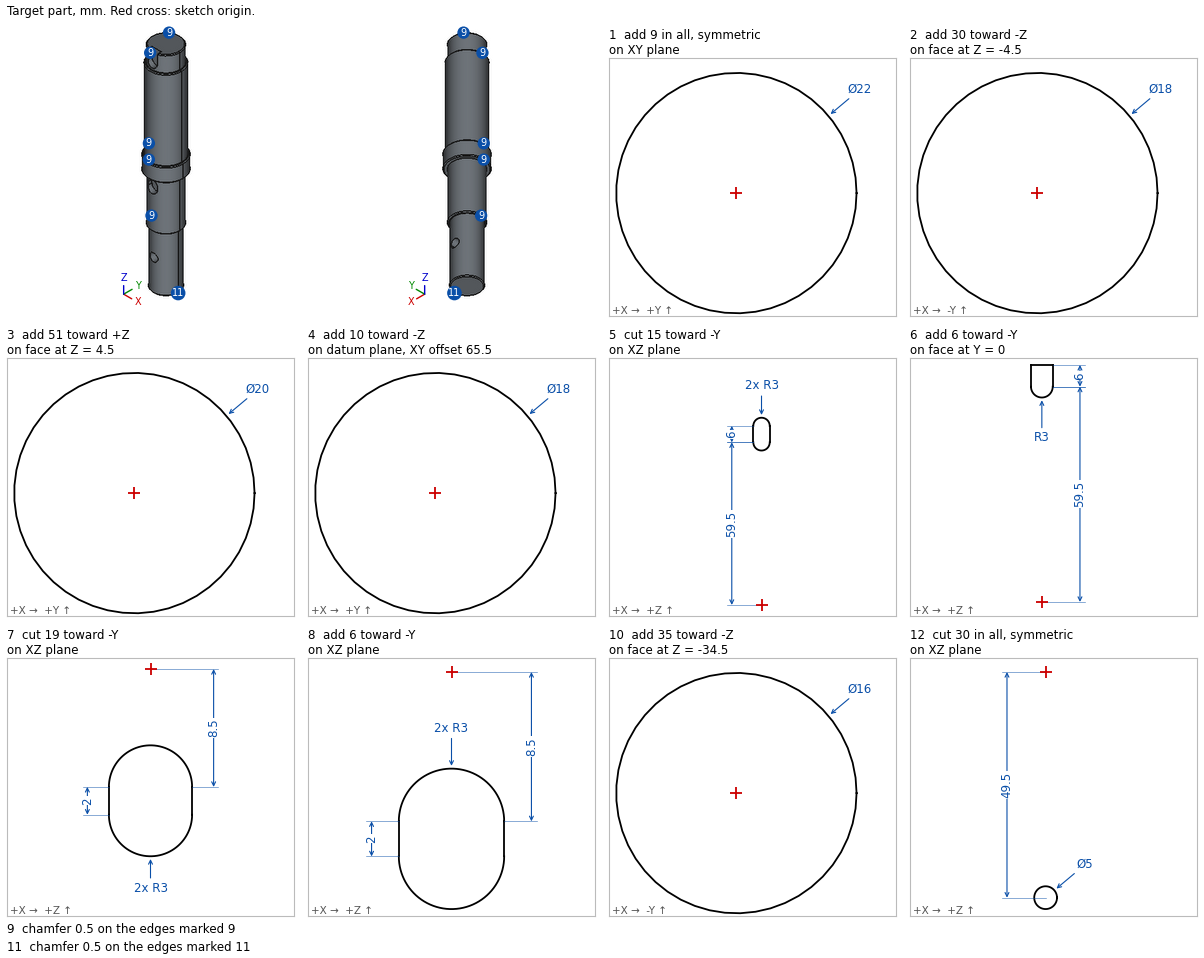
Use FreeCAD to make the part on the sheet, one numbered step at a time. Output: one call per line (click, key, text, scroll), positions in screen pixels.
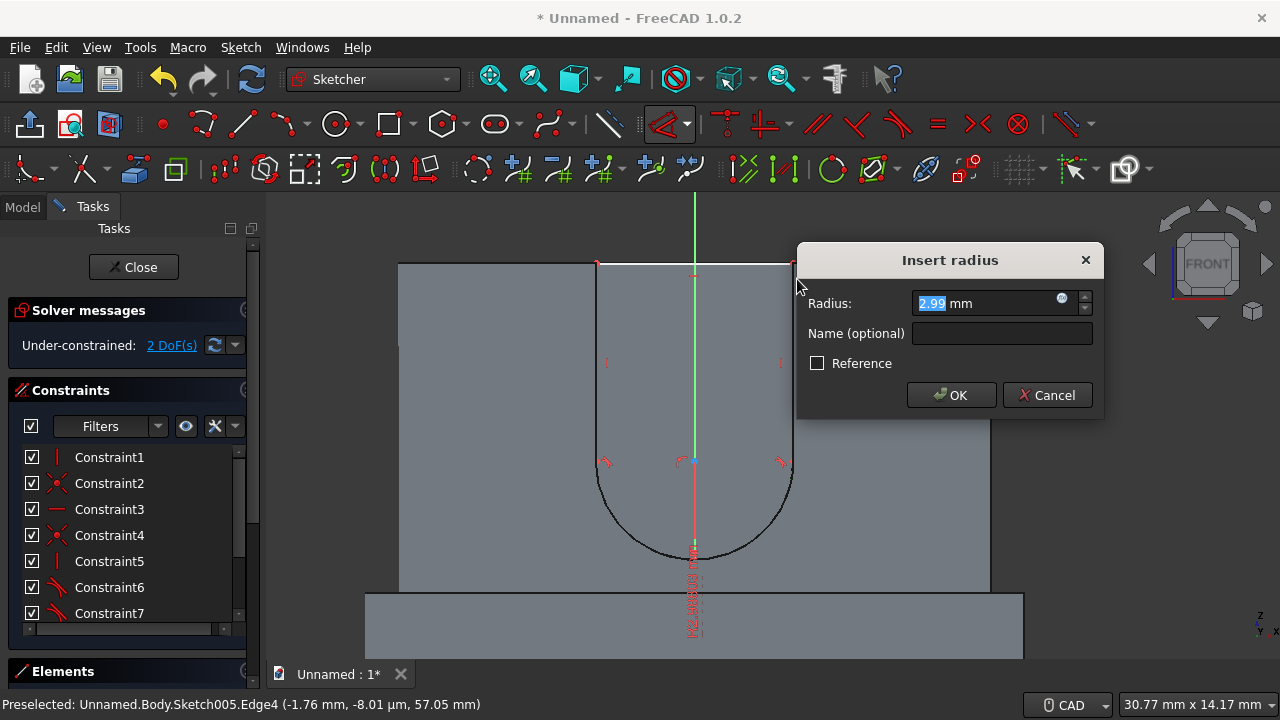
text(3)
key(Return)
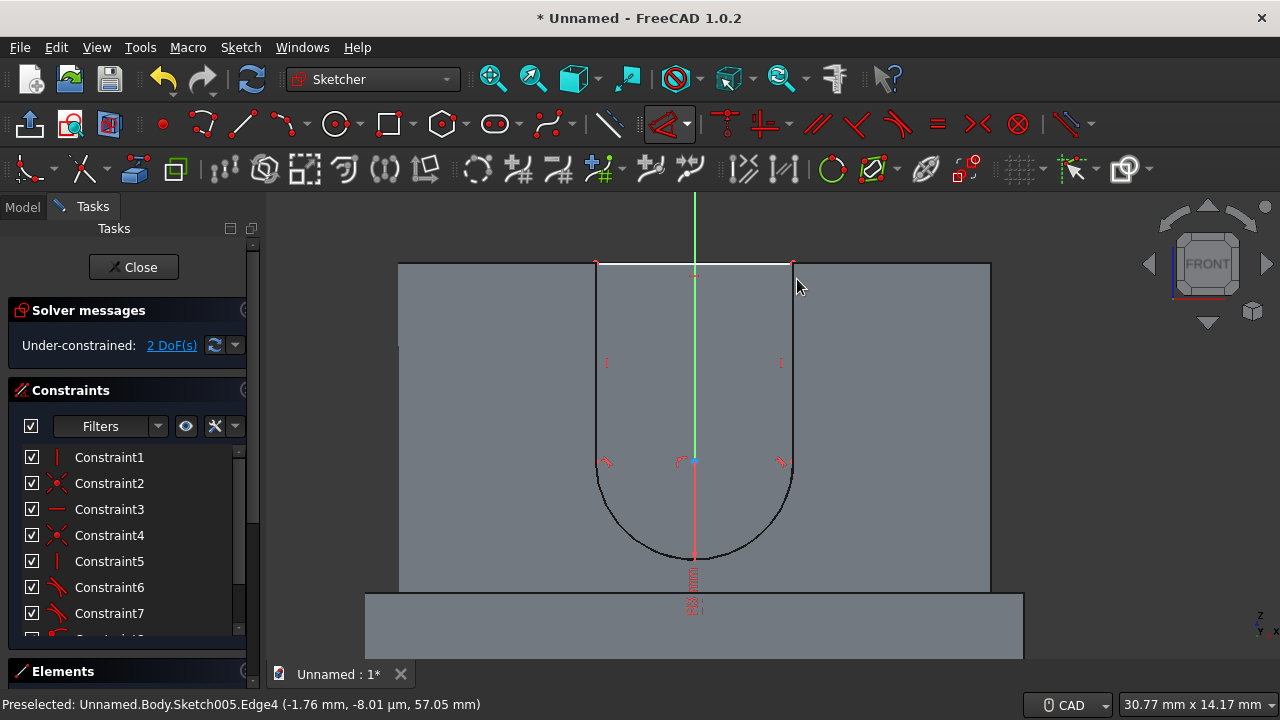
click(793, 403)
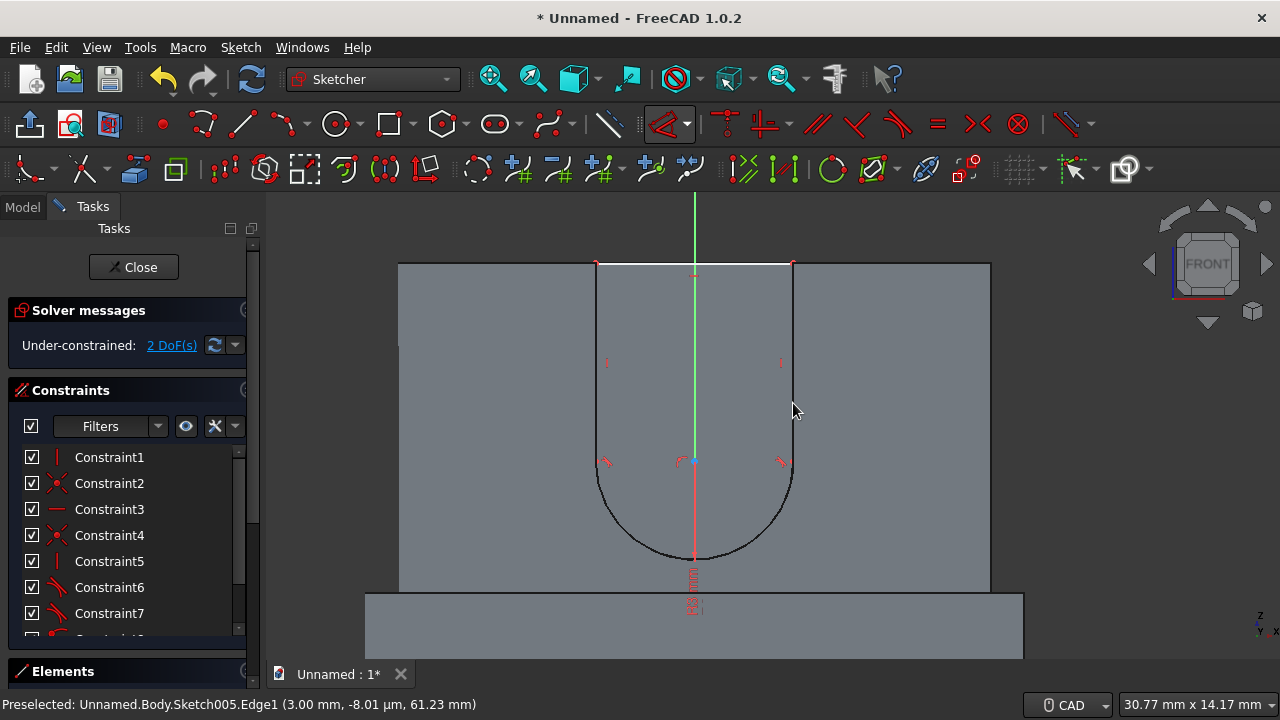
key(i)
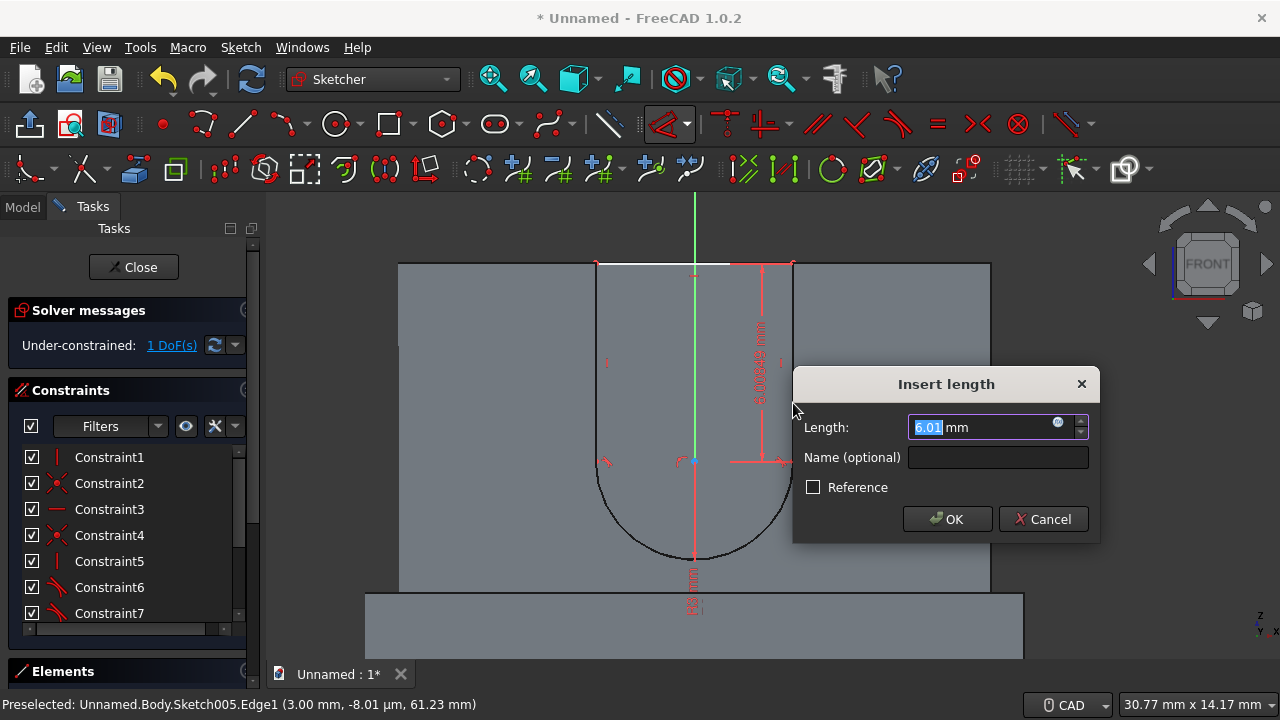
text(6)
key(Return)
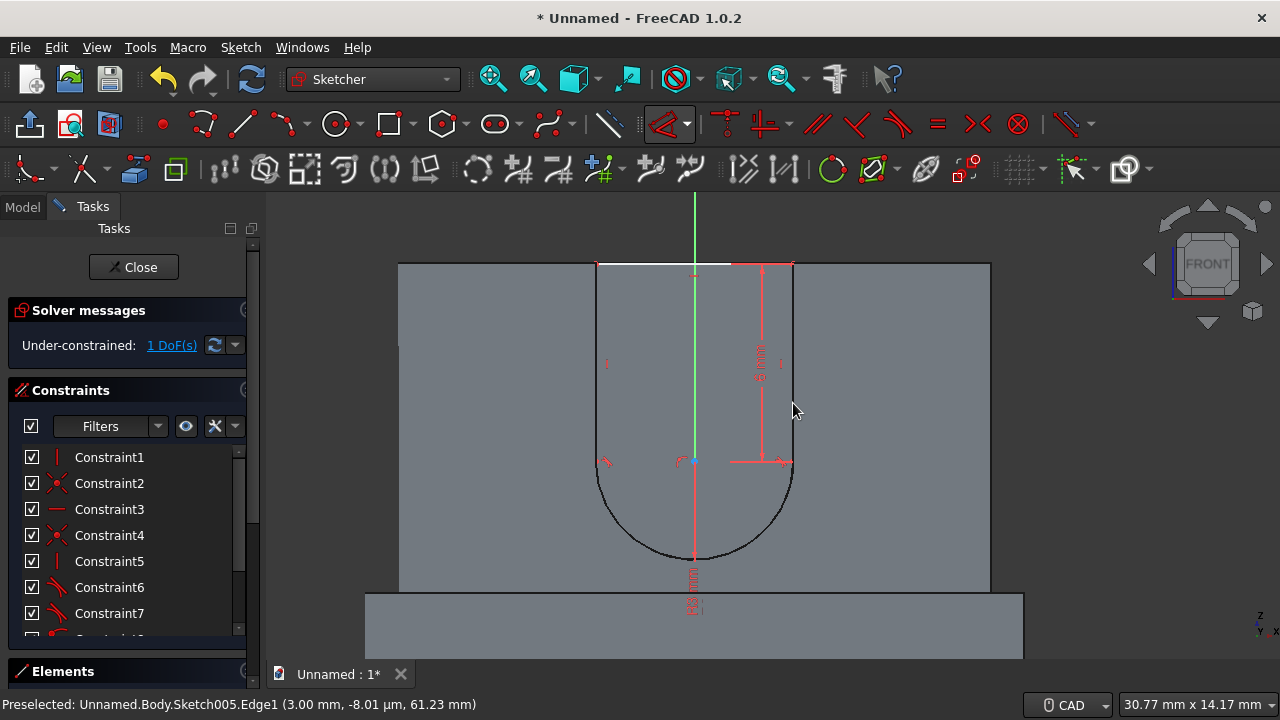
click(793, 462)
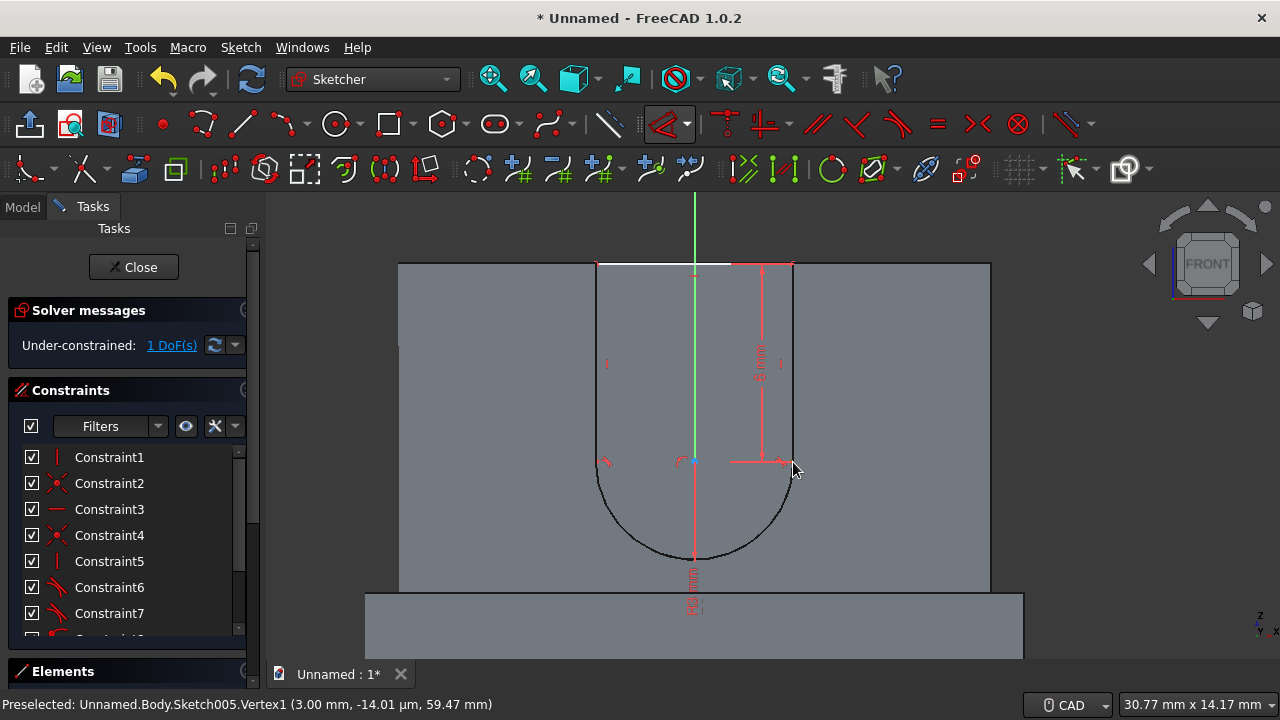
key(i)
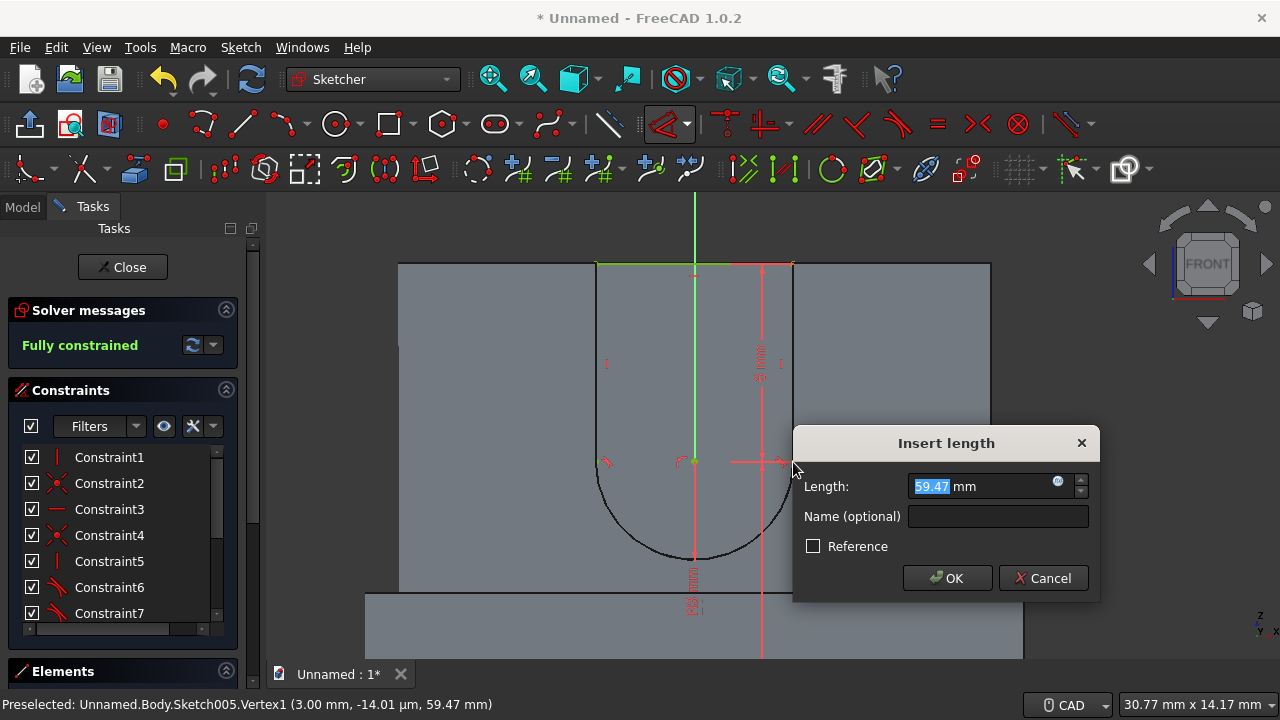
text(59.5)
key(Return)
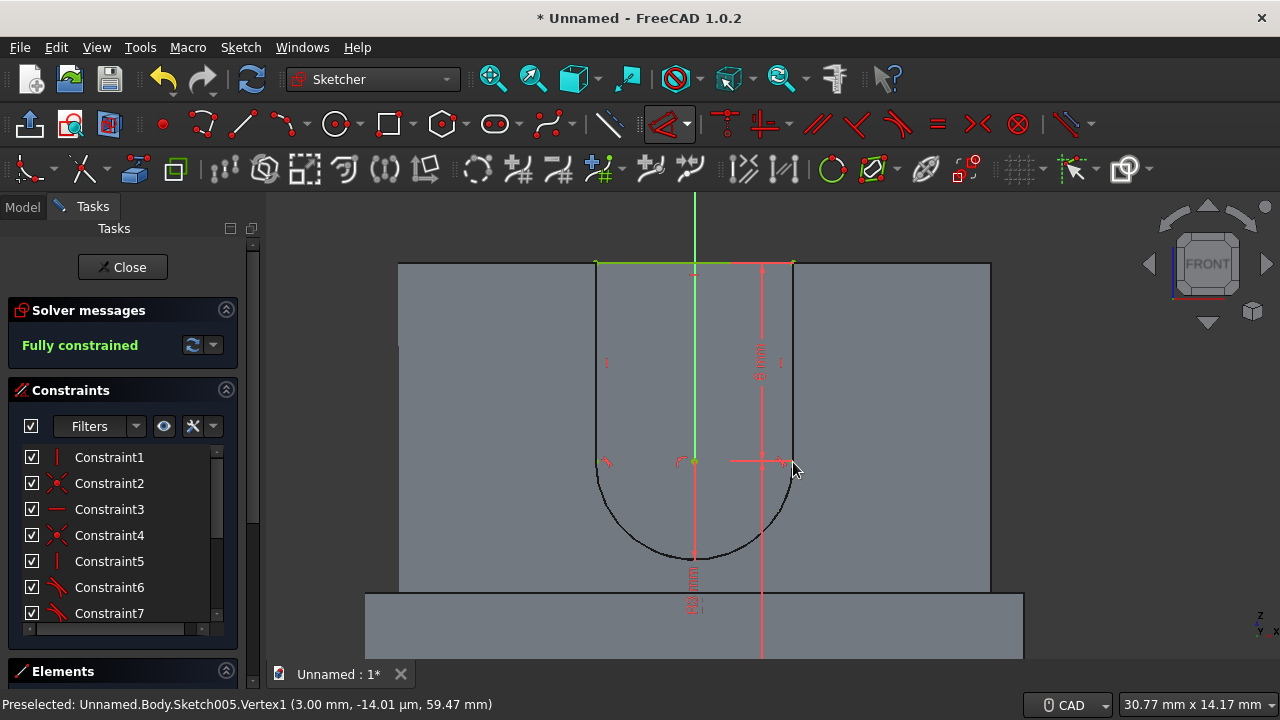
click(123, 267)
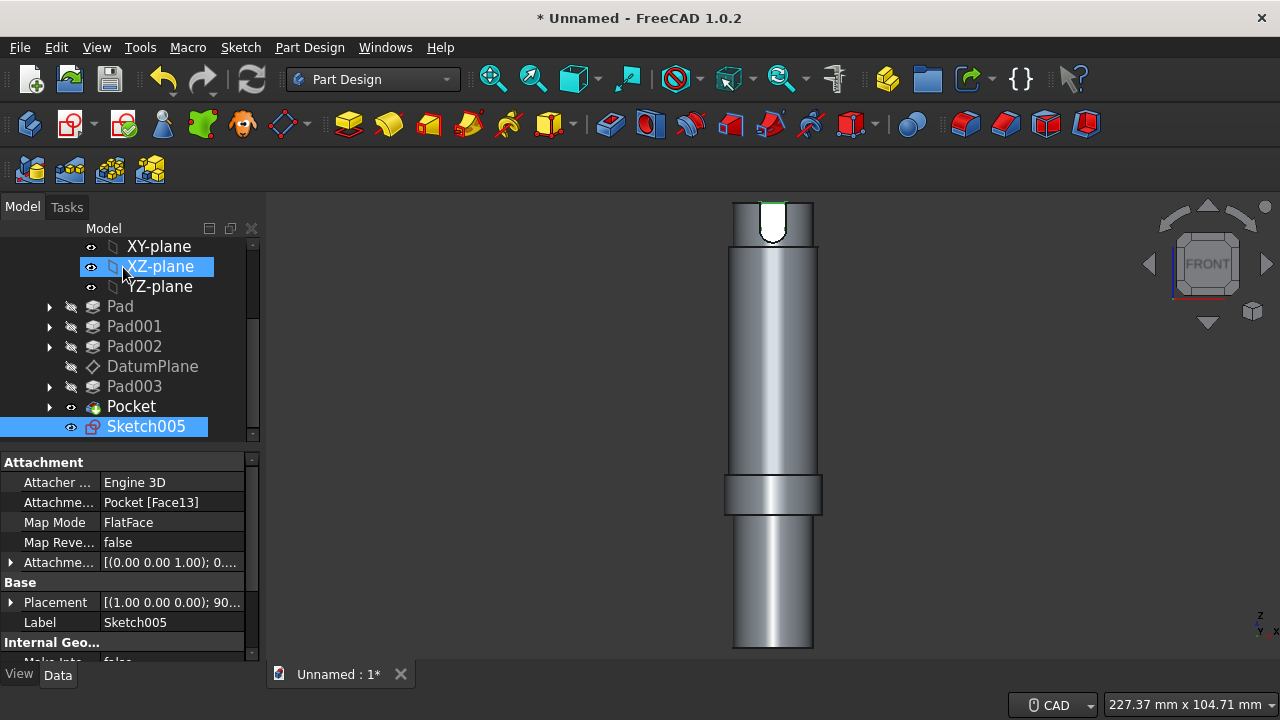
click(350, 124)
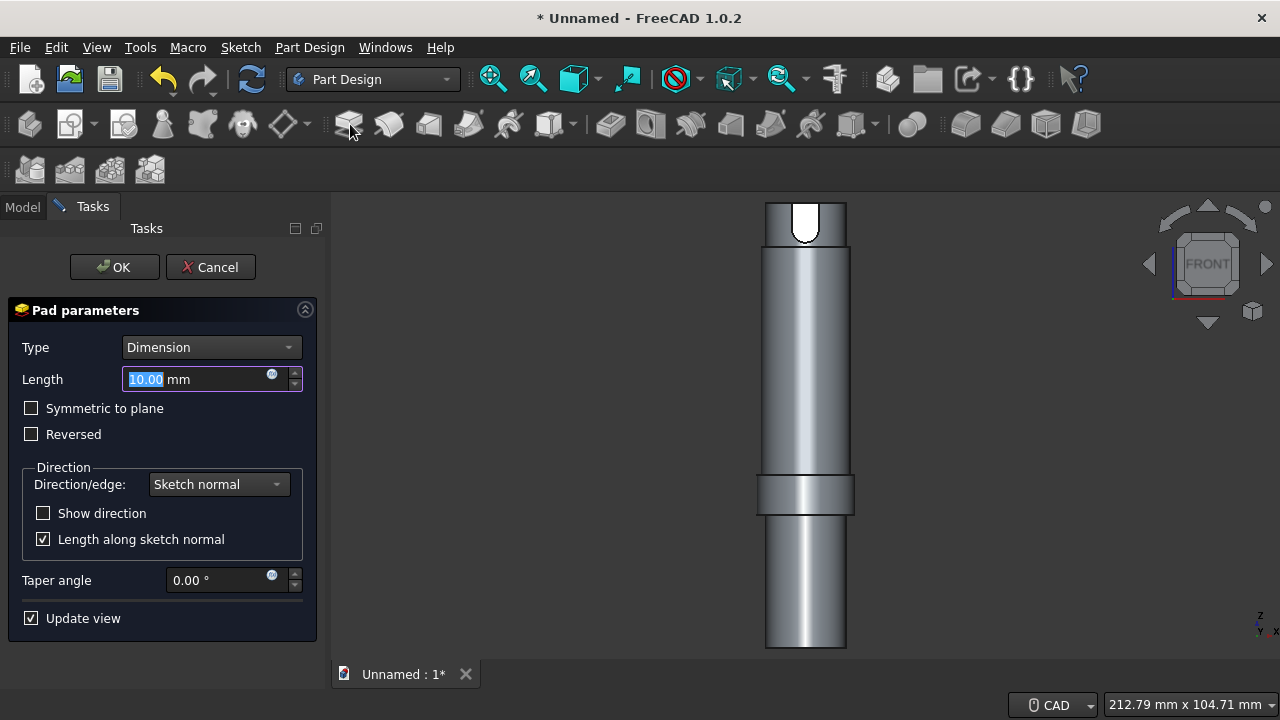
text(6)
key(Tab)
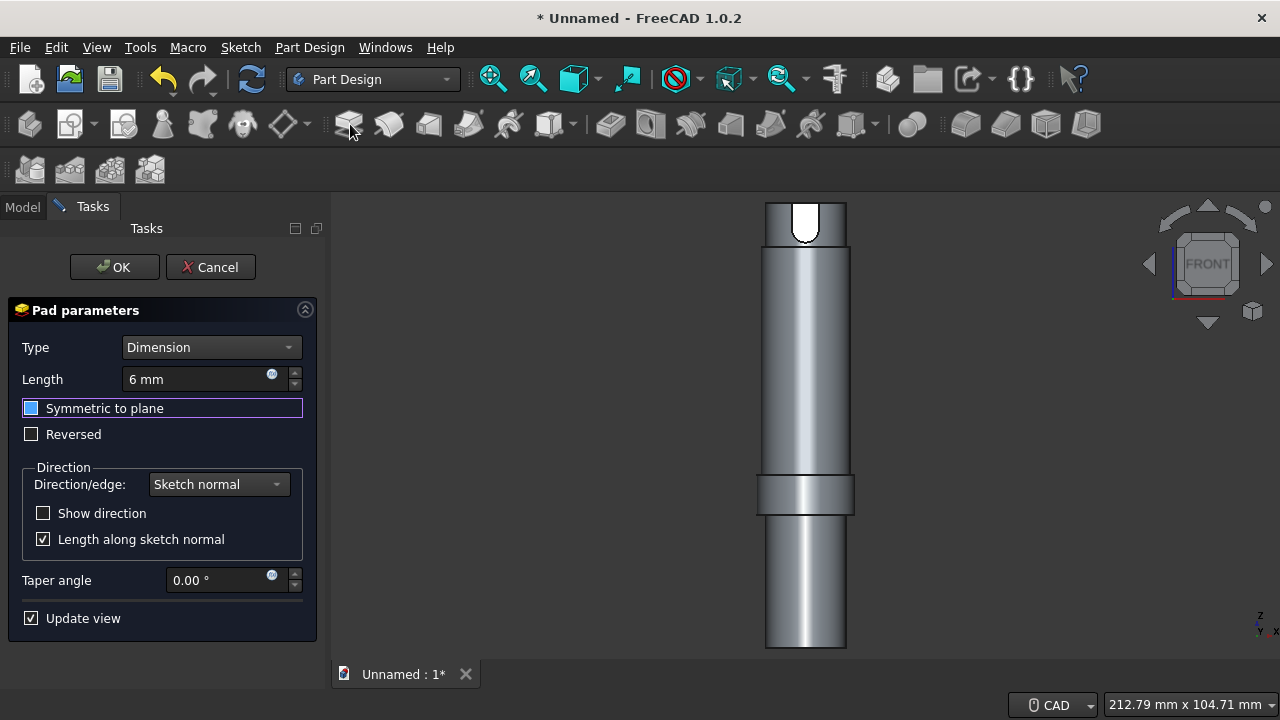
click(115, 267)